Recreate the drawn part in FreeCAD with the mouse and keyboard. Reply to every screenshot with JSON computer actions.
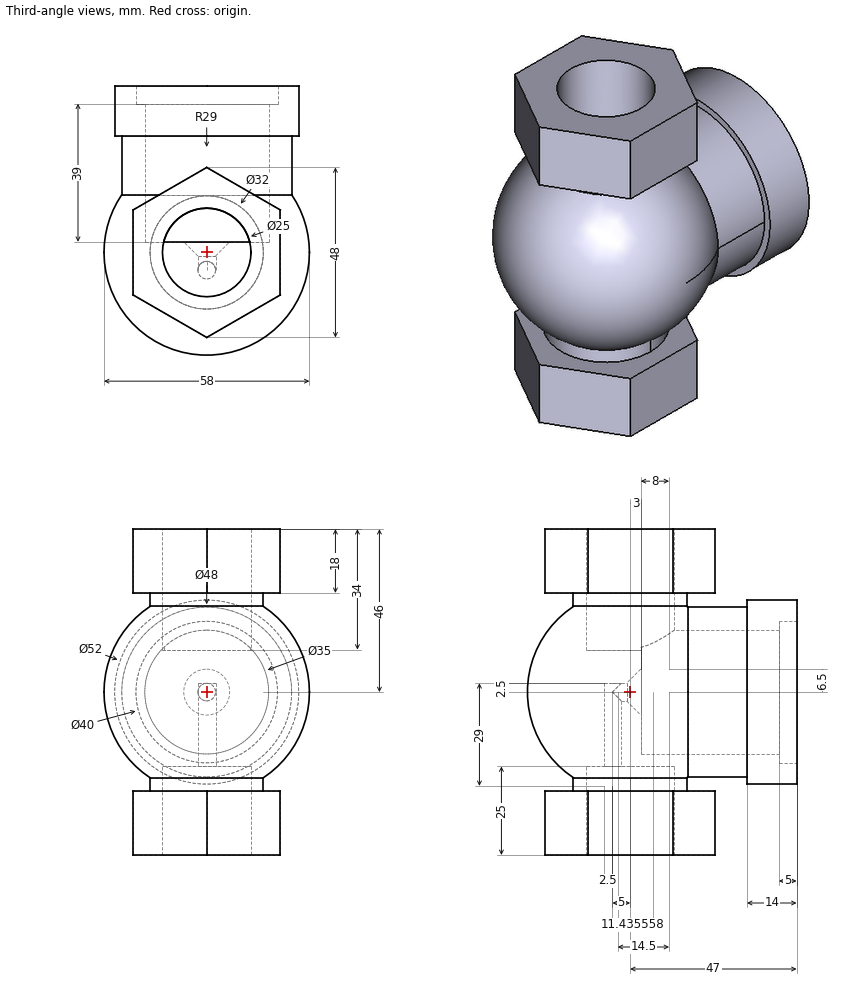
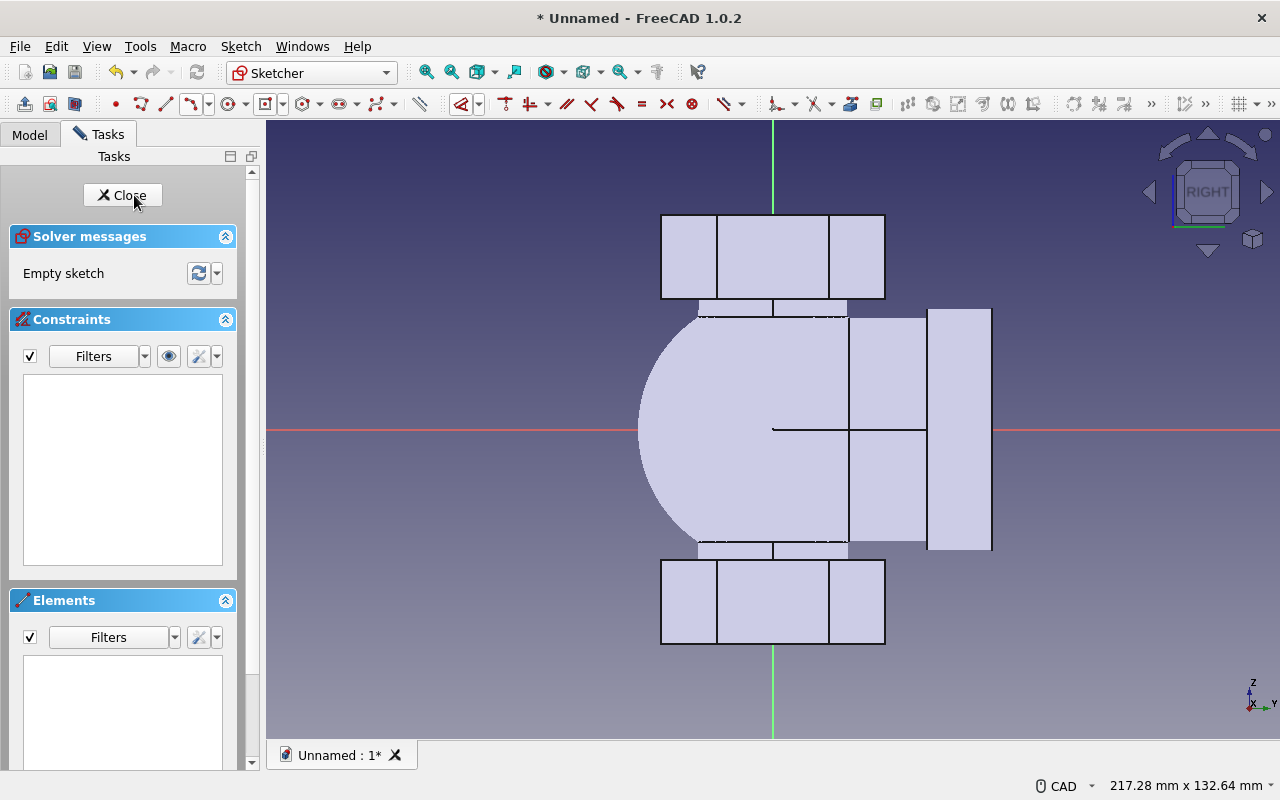
{"action": "left_click", "coordinate": [75, 104]}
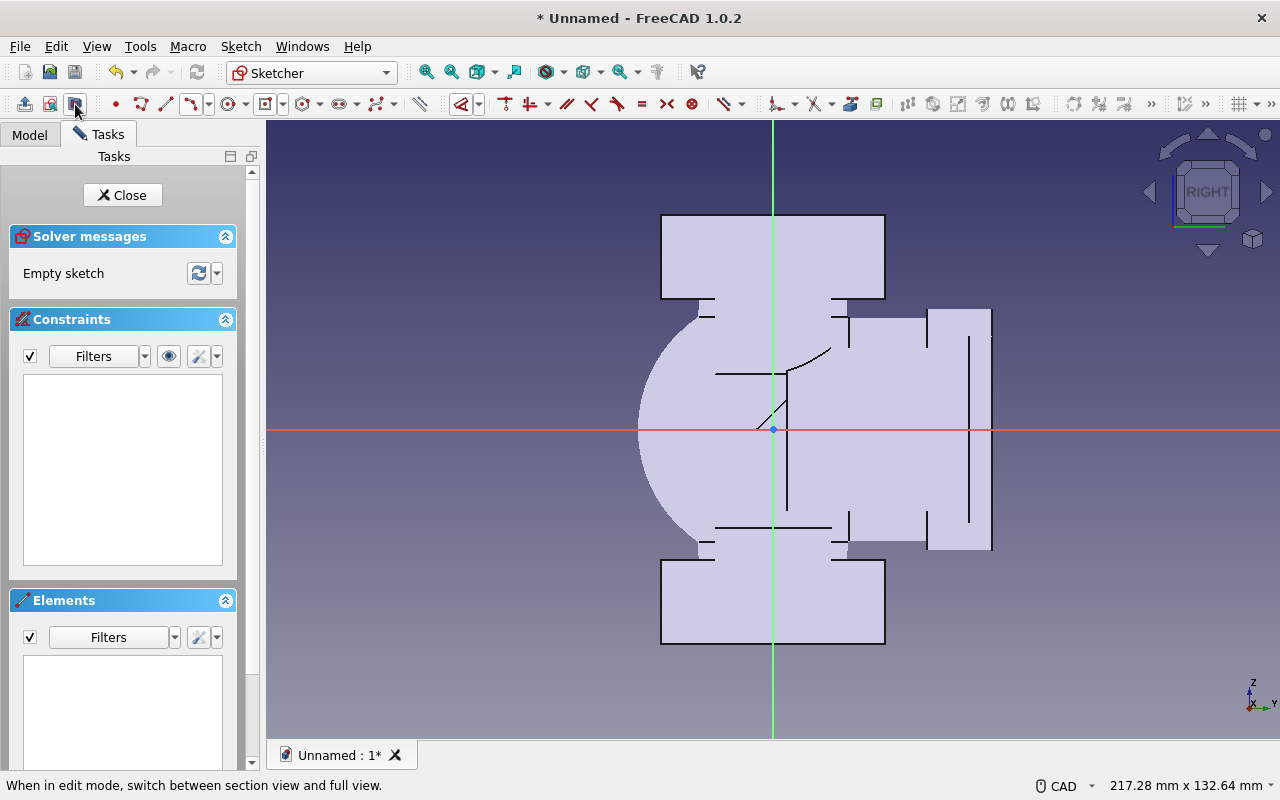
{"action": "scroll", "coordinate": [797, 580], "scroll_direction": "up", "scroll_amount": 4}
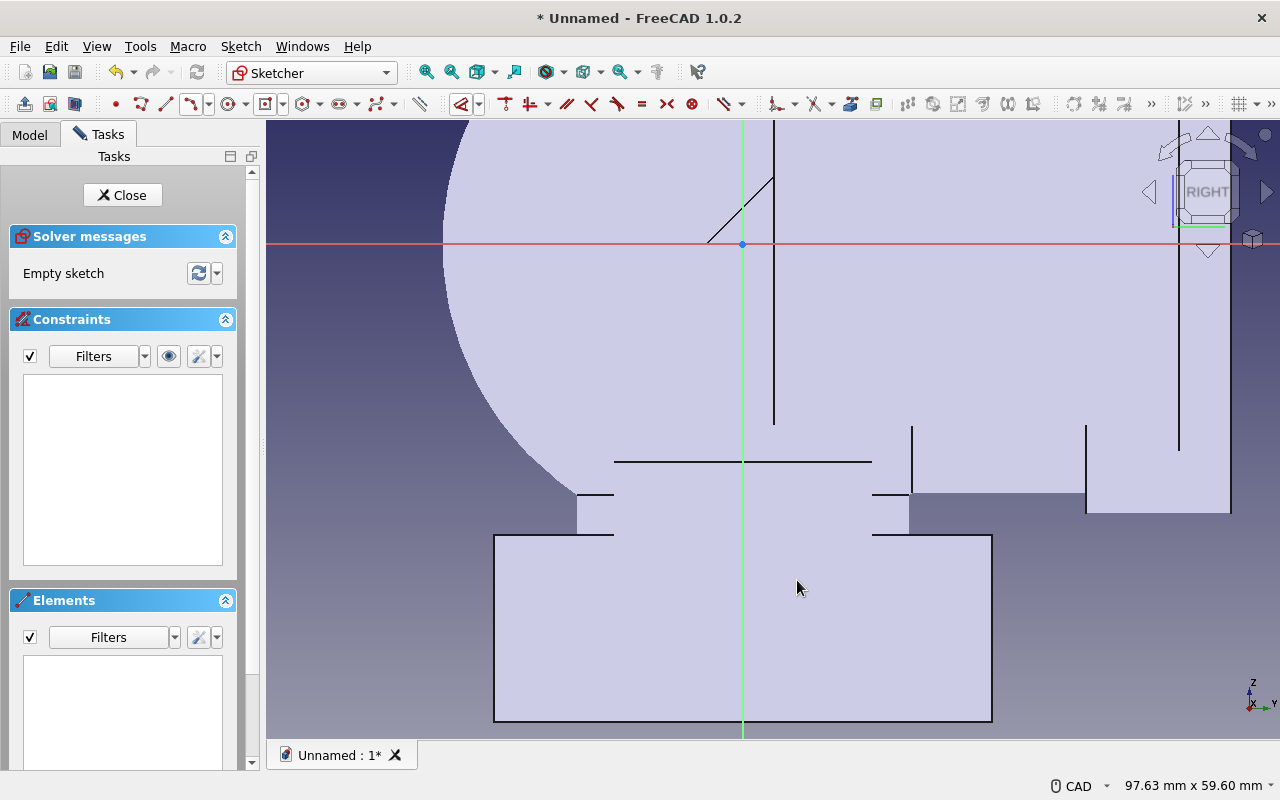
{"action": "key", "text": "g r"}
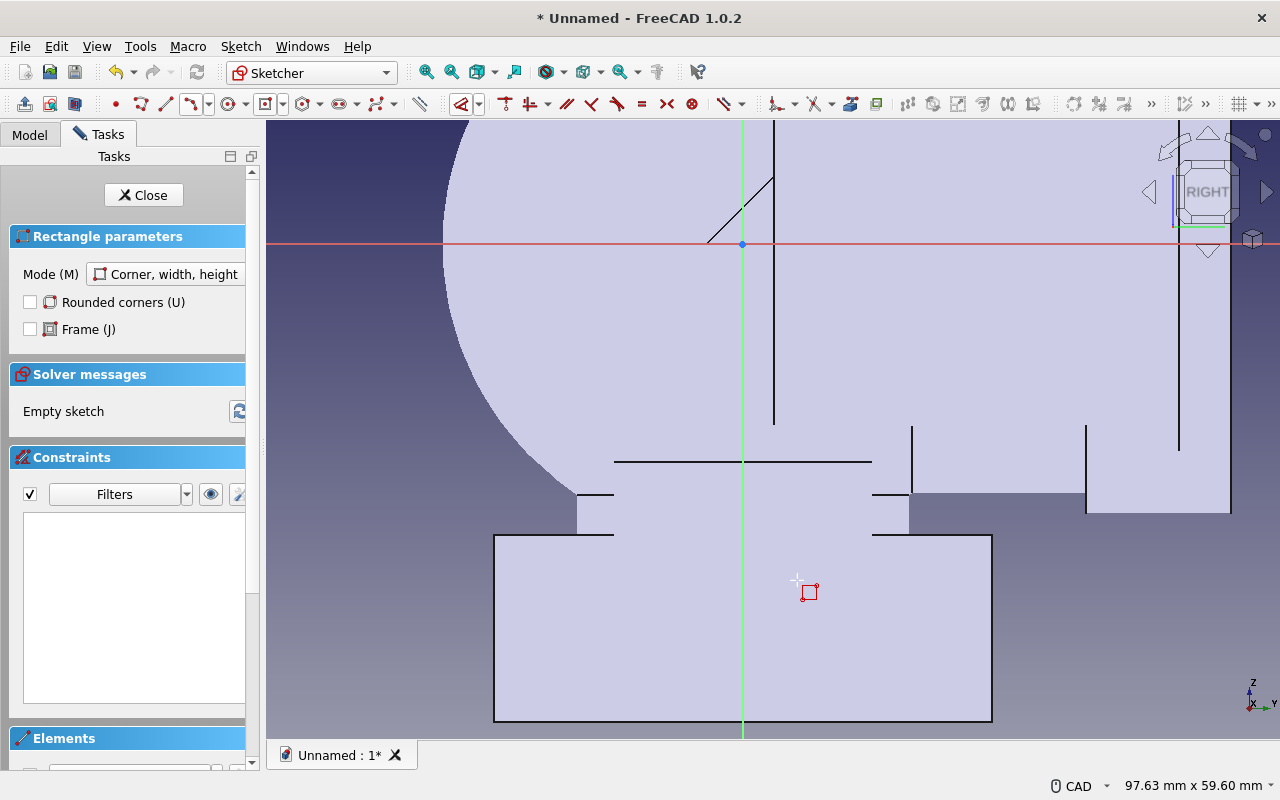
{"action": "left_click", "coordinate": [665, 218]}
{"action": "left_click", "coordinate": [691, 519]}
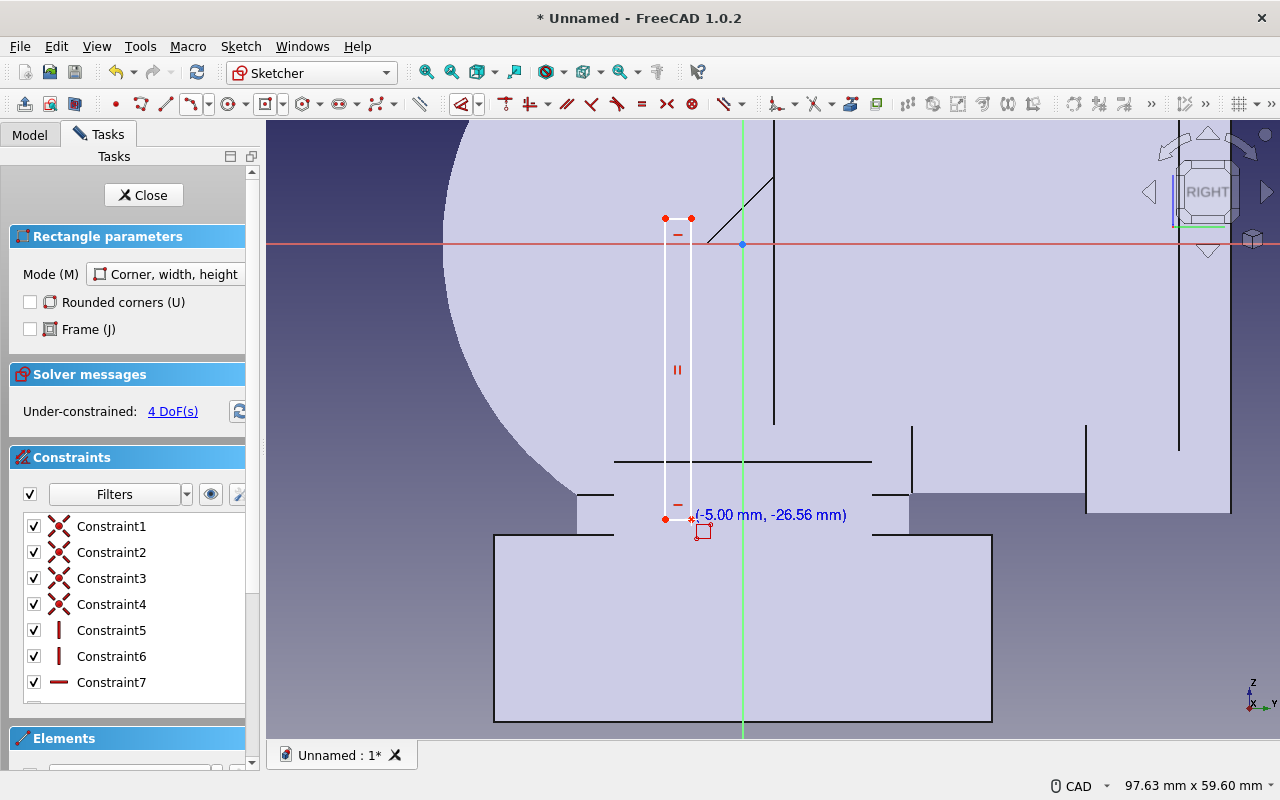
{"action": "left_click", "coordinate": [166, 104]}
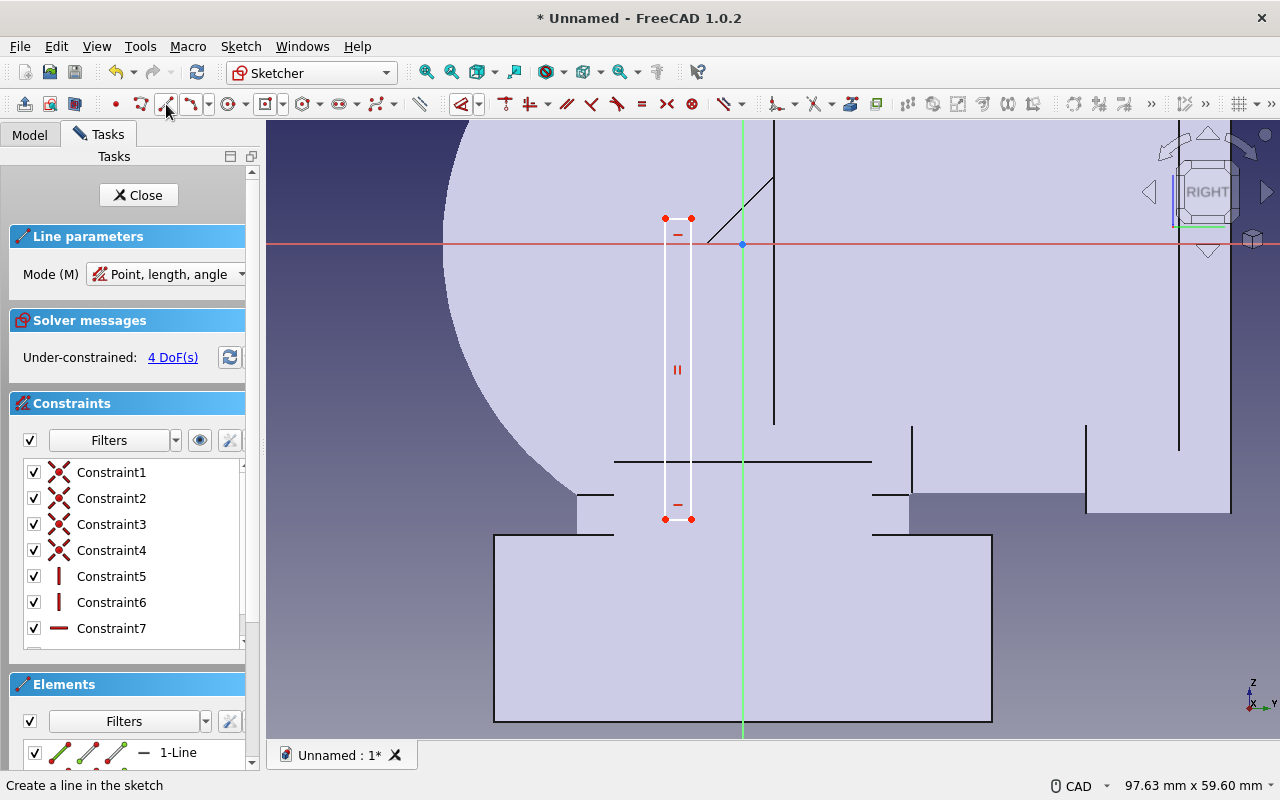
{"action": "left_click", "coordinate": [691, 549]}
{"action": "left_click", "coordinate": [691, 640]}
{"action": "key", "text": "Escape"}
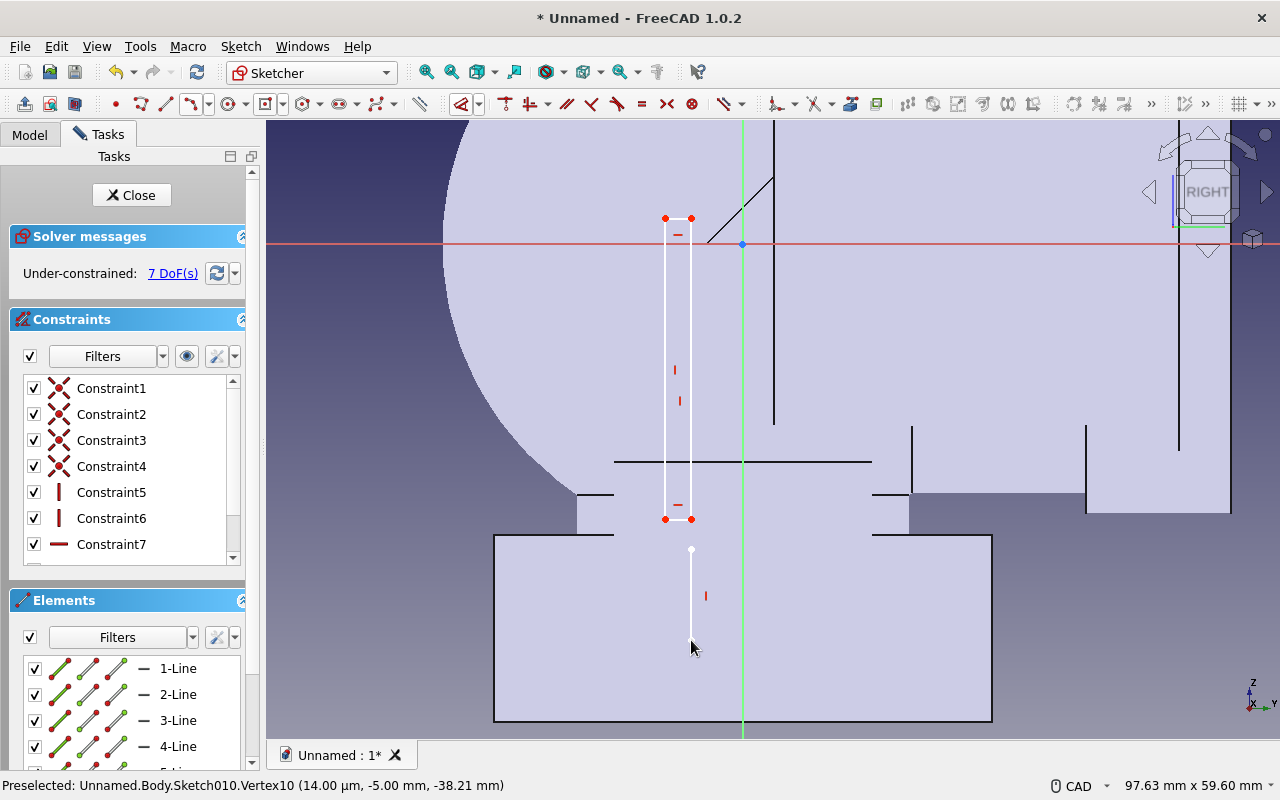
{"action": "left_click", "coordinate": [691, 577]}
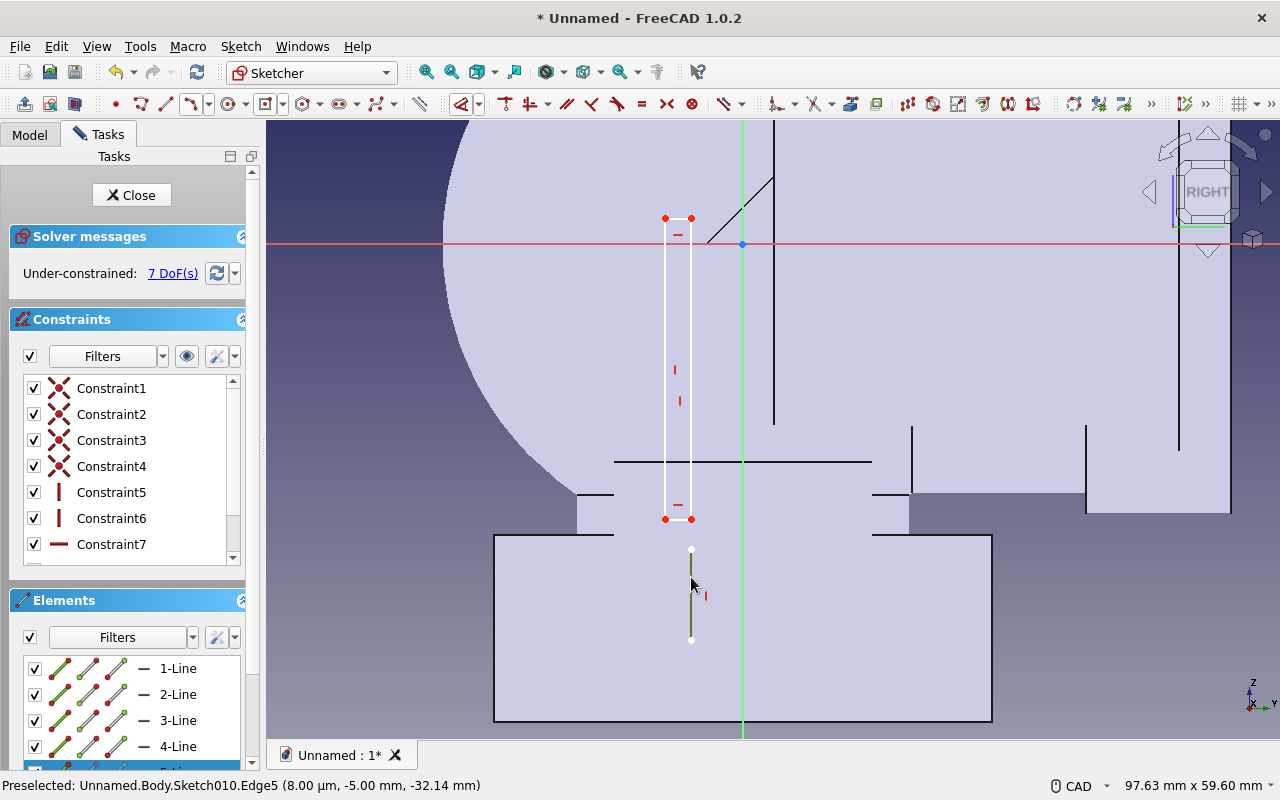
{"action": "left_click", "coordinate": [420, 104]}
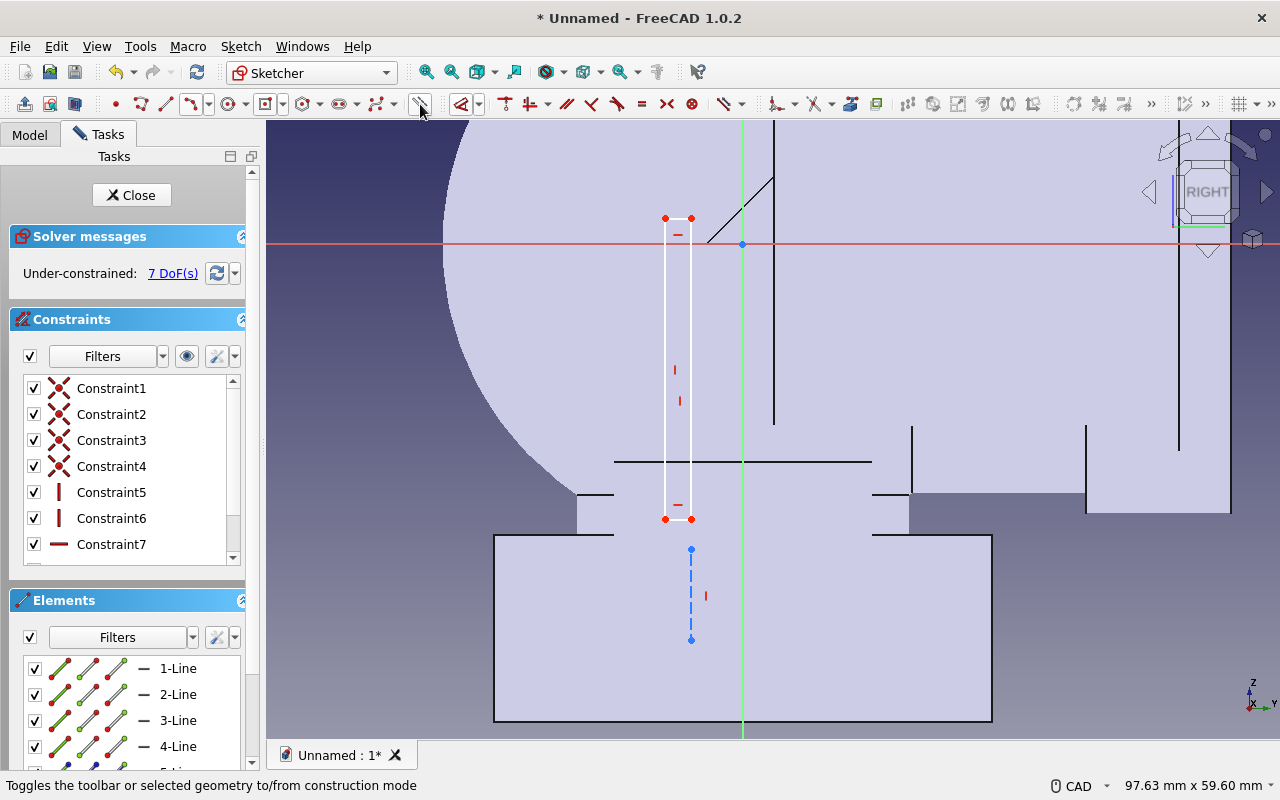
{"action": "left_click", "coordinate": [665, 309]}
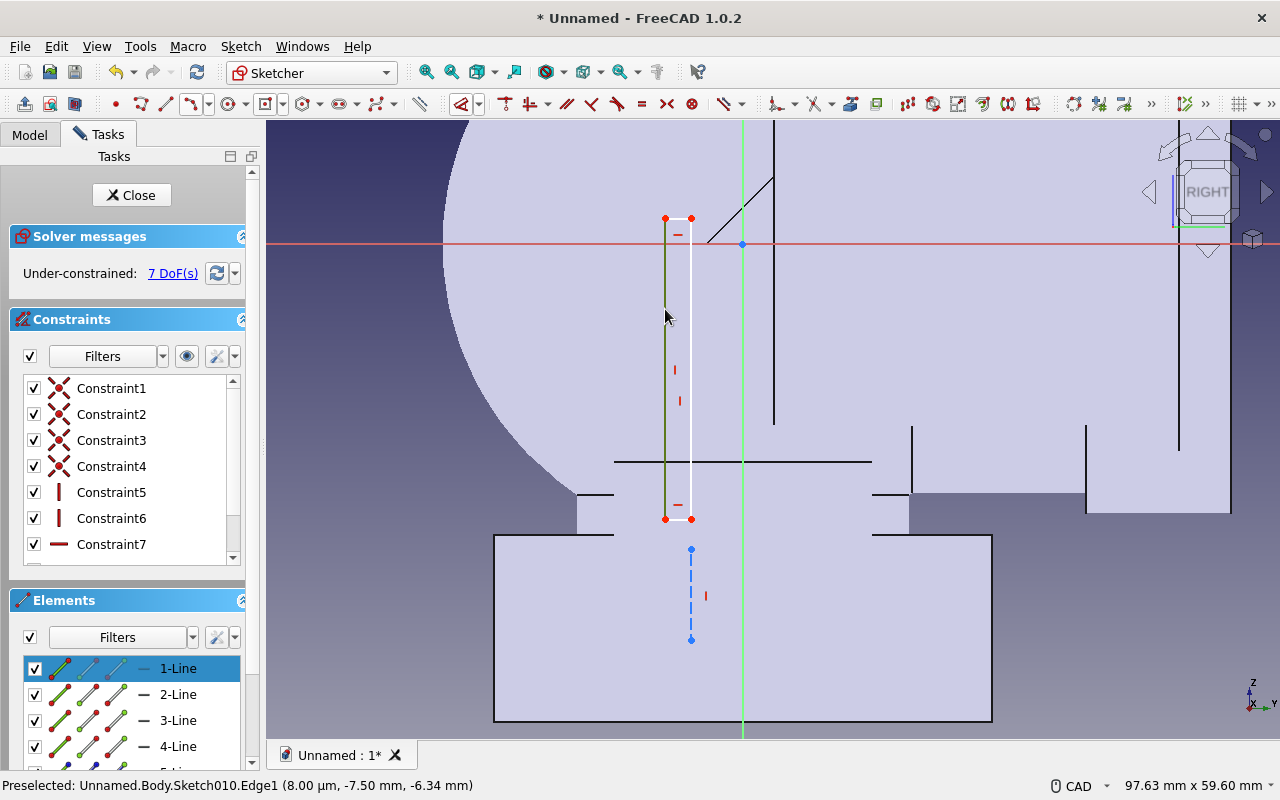
{"action": "key", "text": "i"}